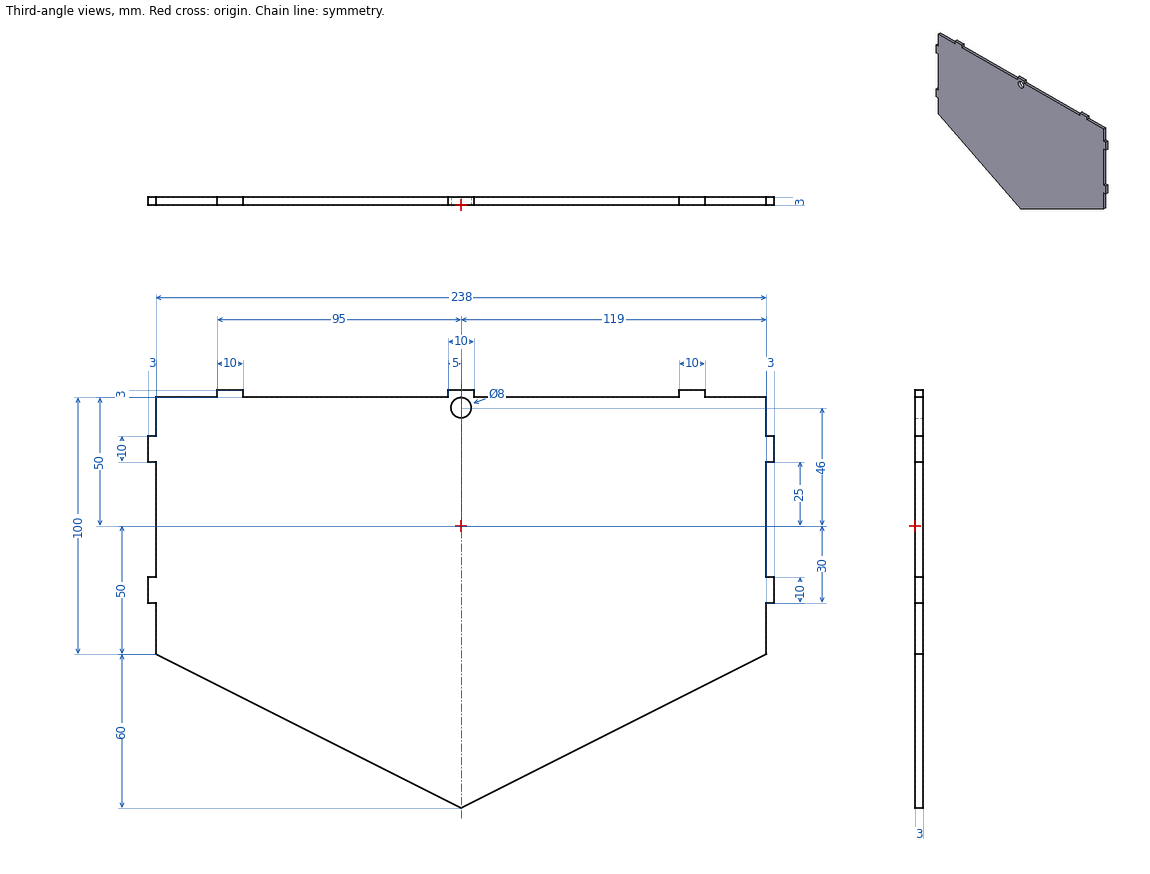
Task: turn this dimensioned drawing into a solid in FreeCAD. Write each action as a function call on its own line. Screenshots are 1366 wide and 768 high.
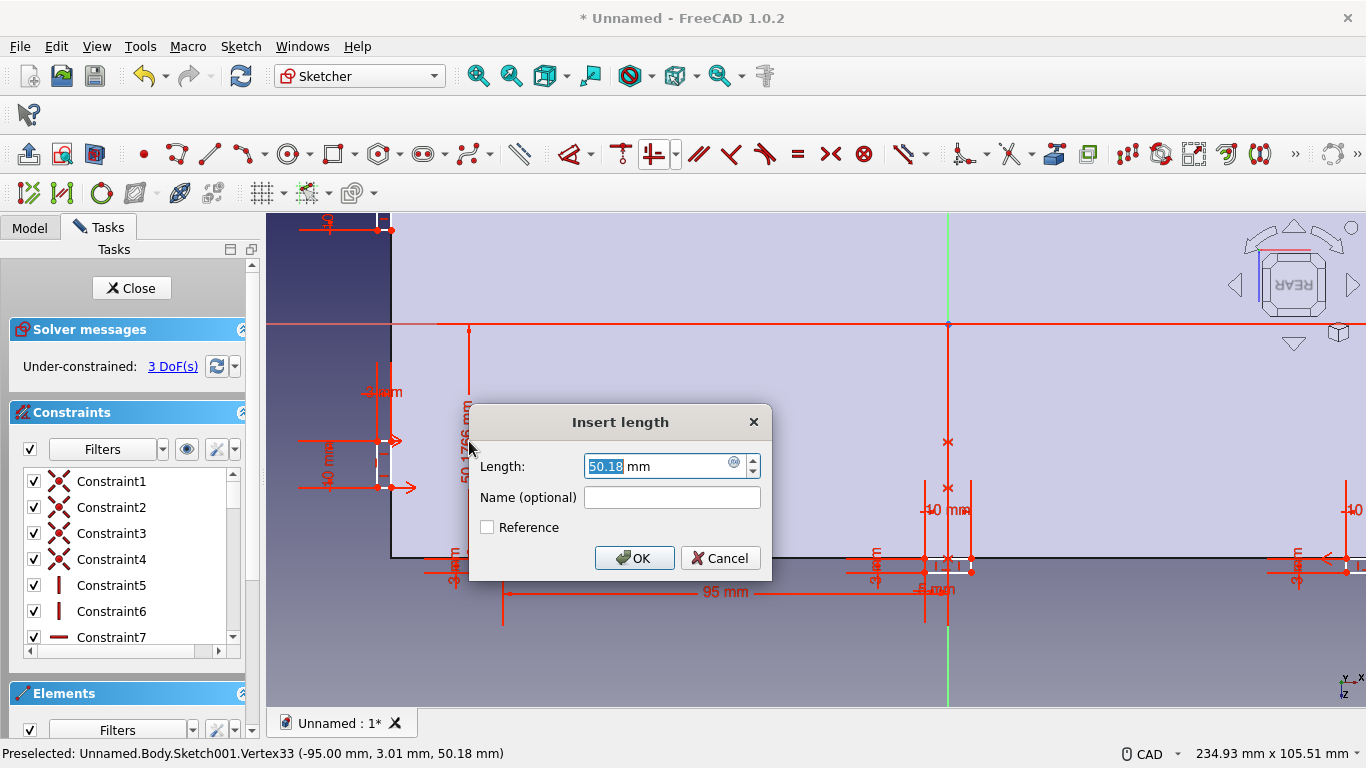
text(50)
key(Return)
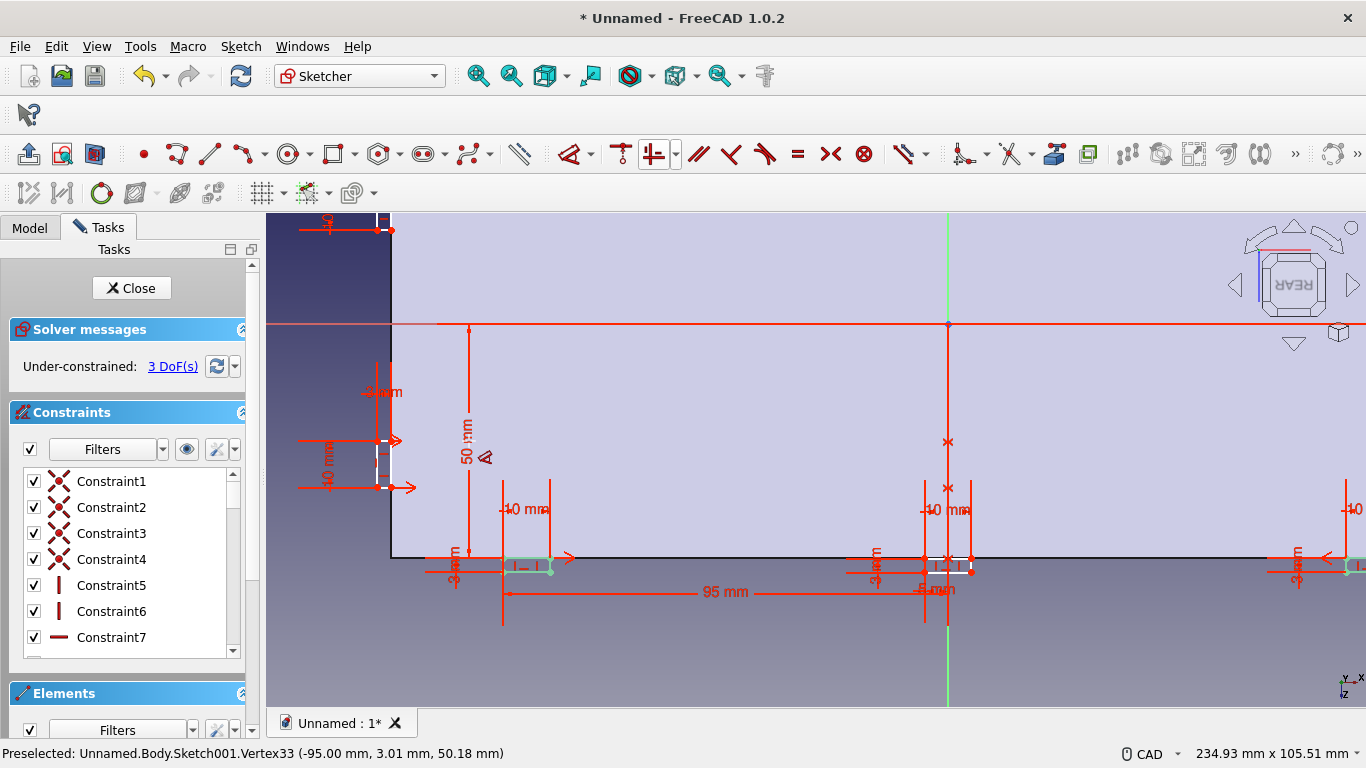
click(925, 559)
click(891, 441)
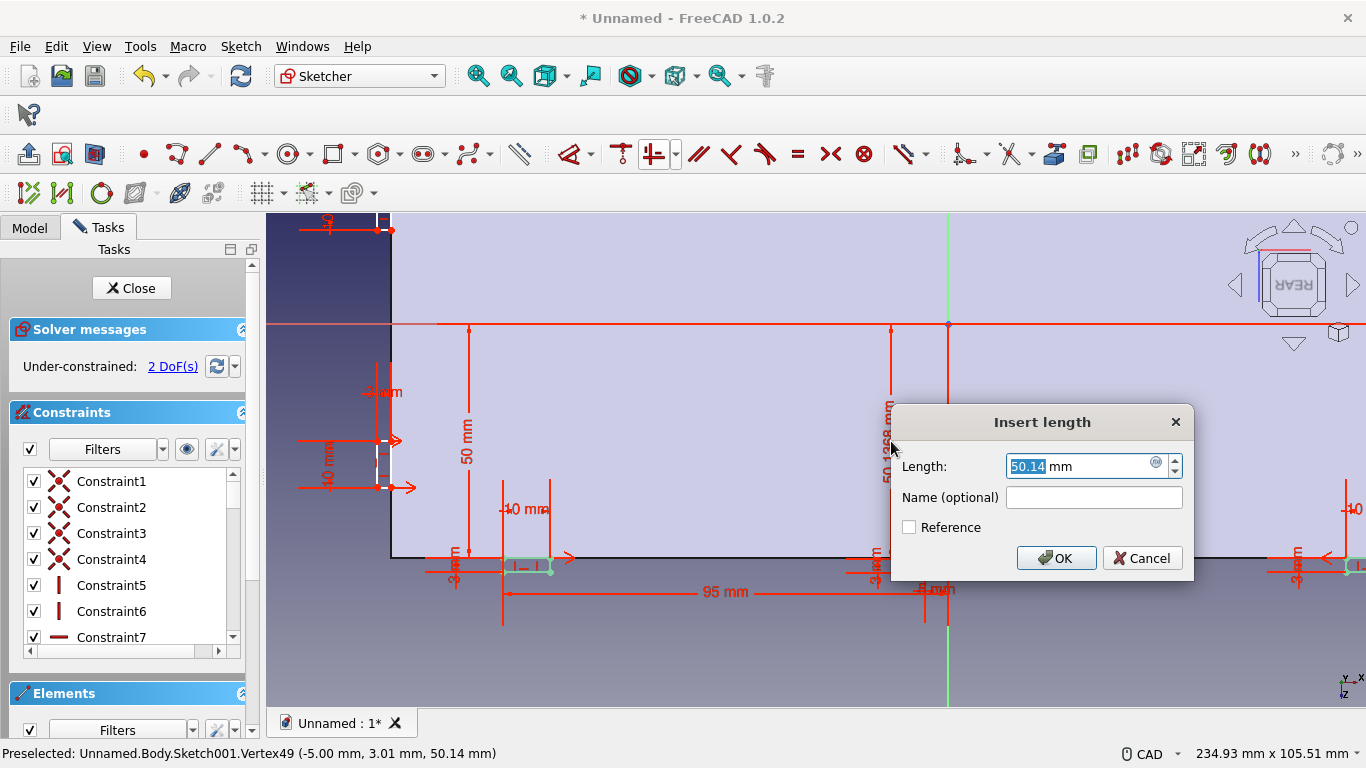
text(50)
key(Return)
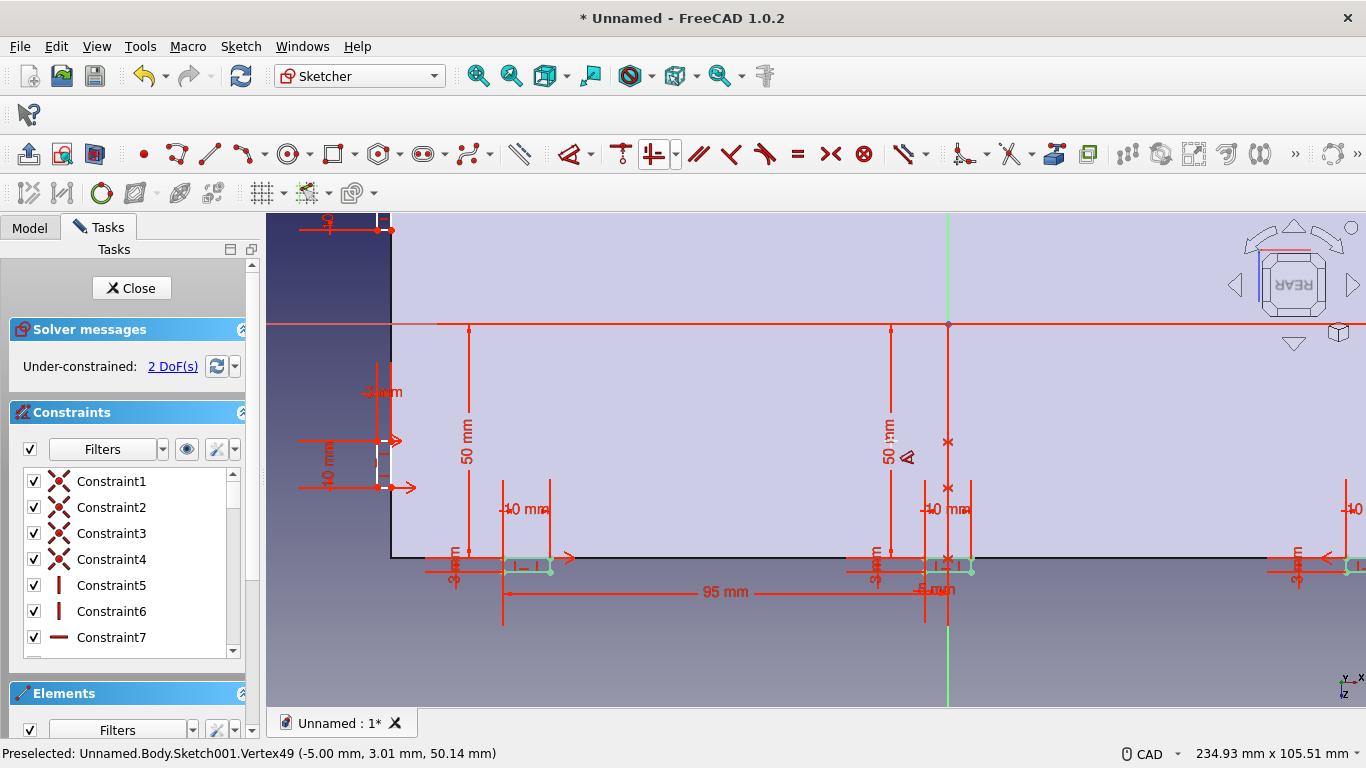
scroll(504, 560, down, 3)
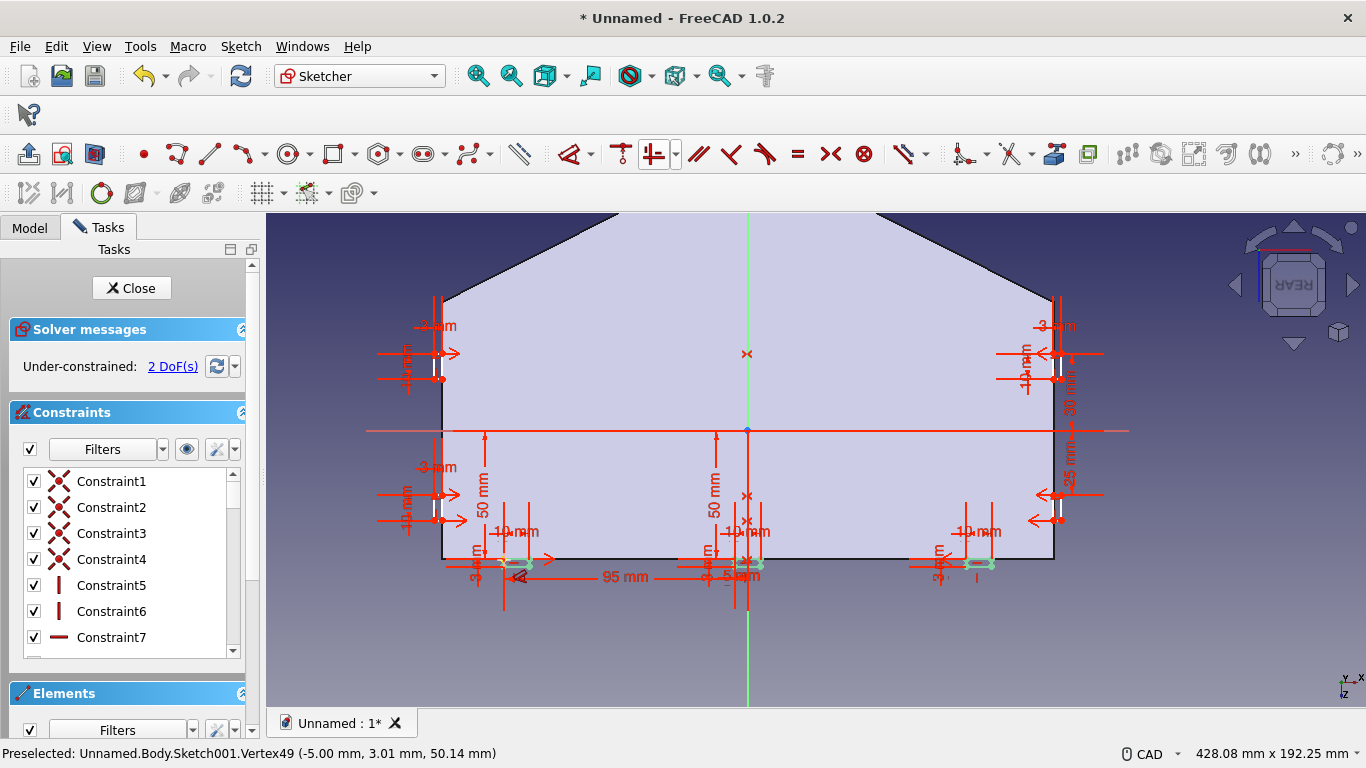
scroll(1053, 354, up, 3)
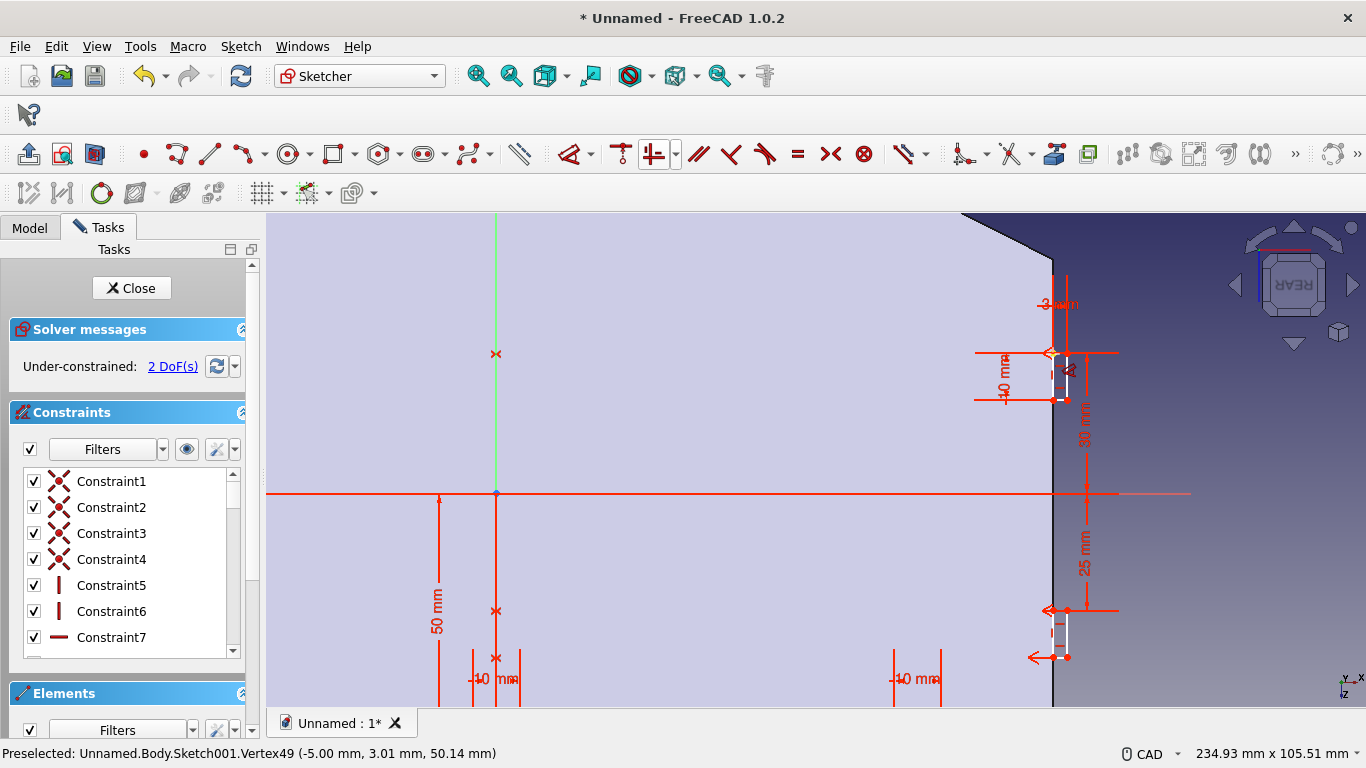
click(1053, 353)
click(775, 319)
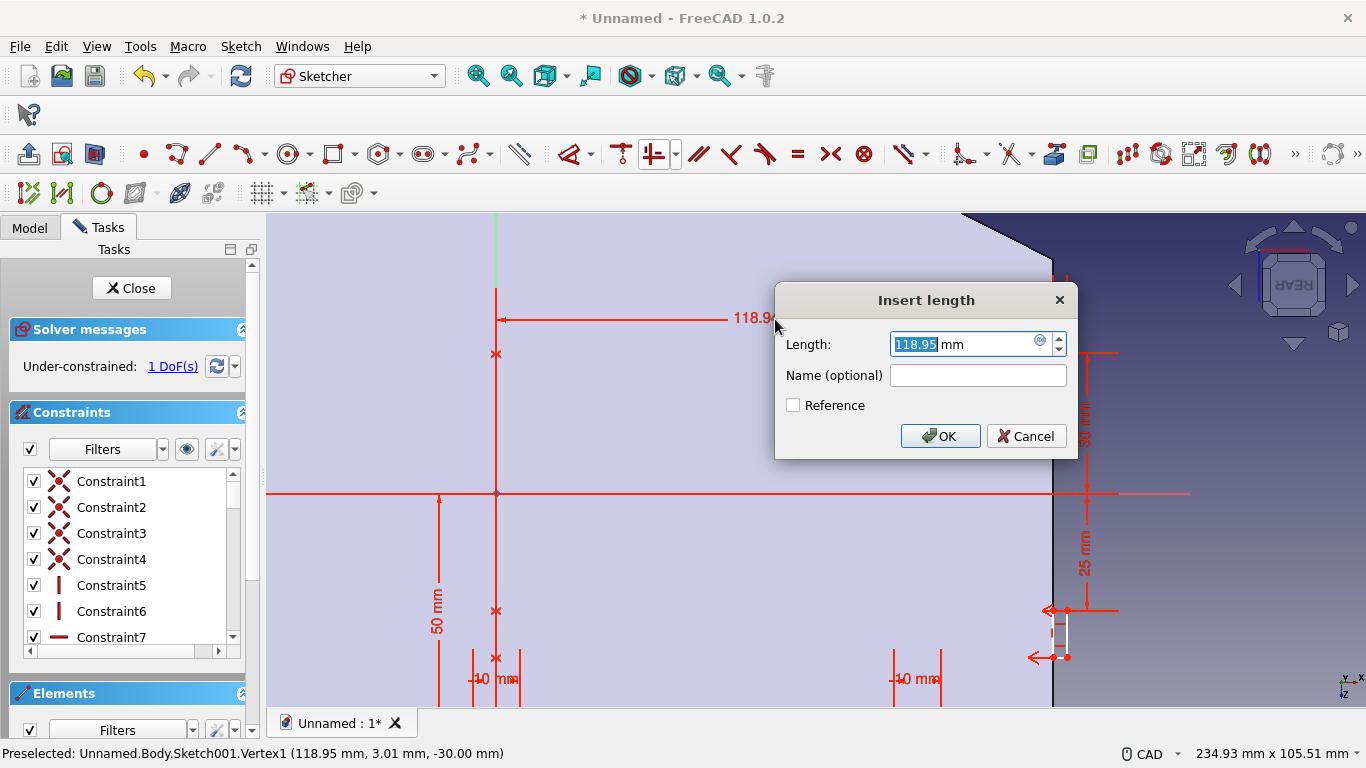
text(119)
key(Return)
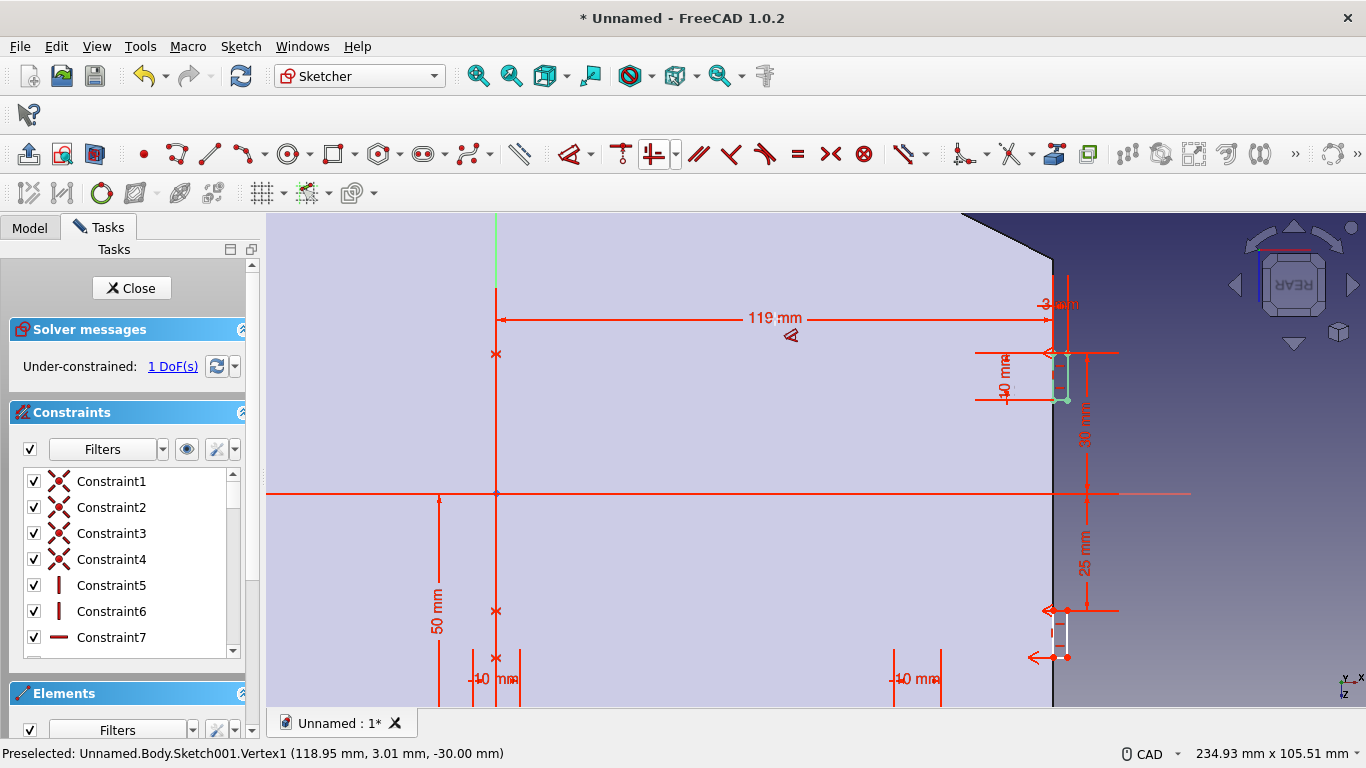
click(1053, 611)
click(775, 645)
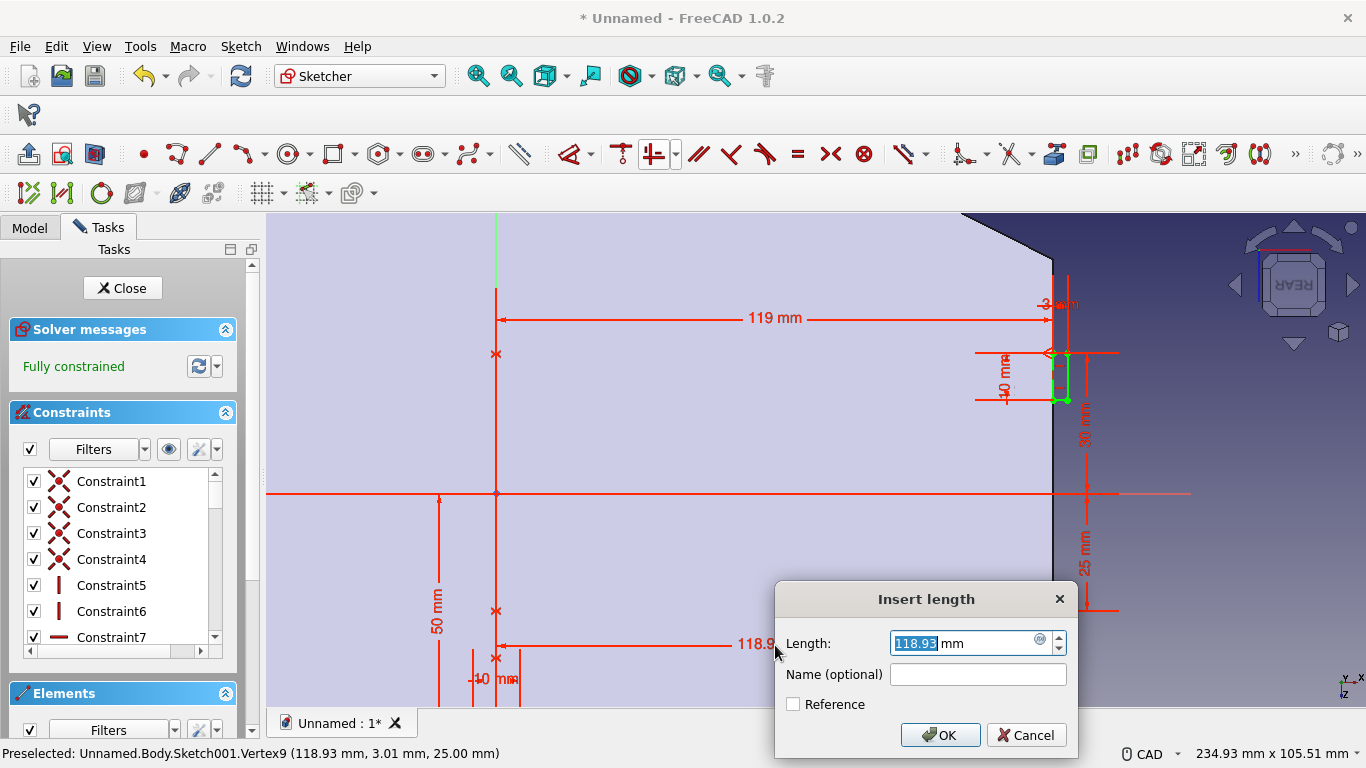
text(119)
key(Return)
key(Escape)